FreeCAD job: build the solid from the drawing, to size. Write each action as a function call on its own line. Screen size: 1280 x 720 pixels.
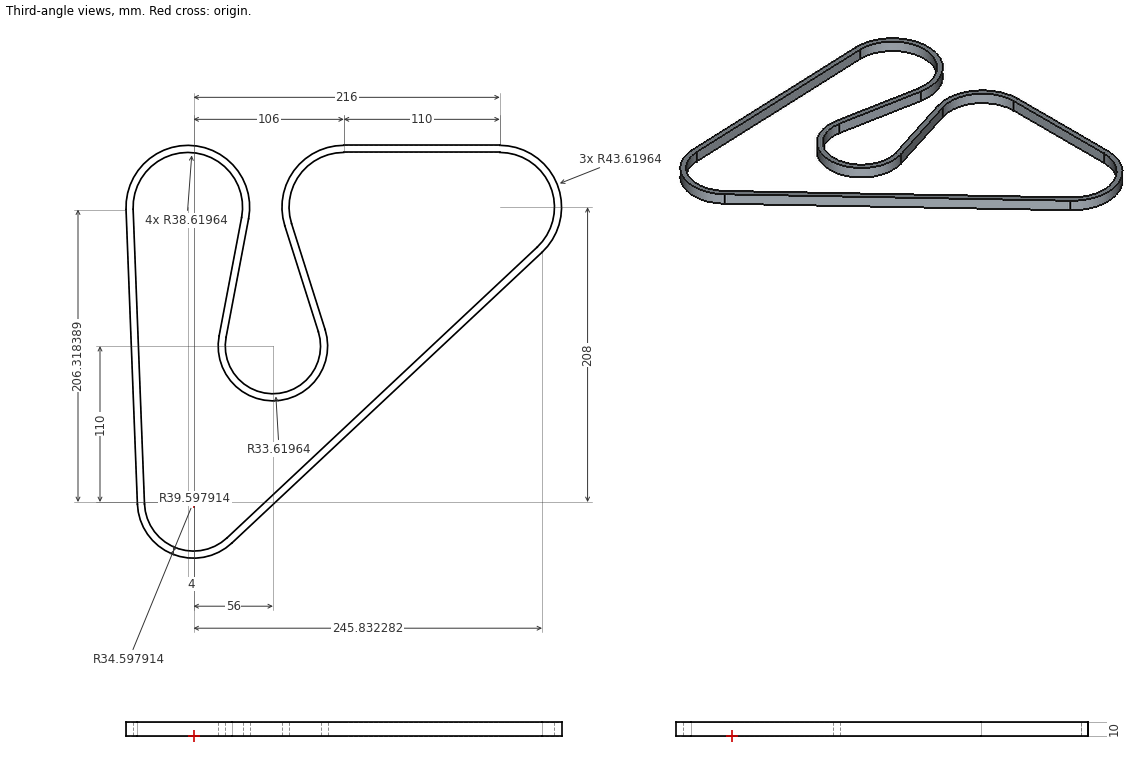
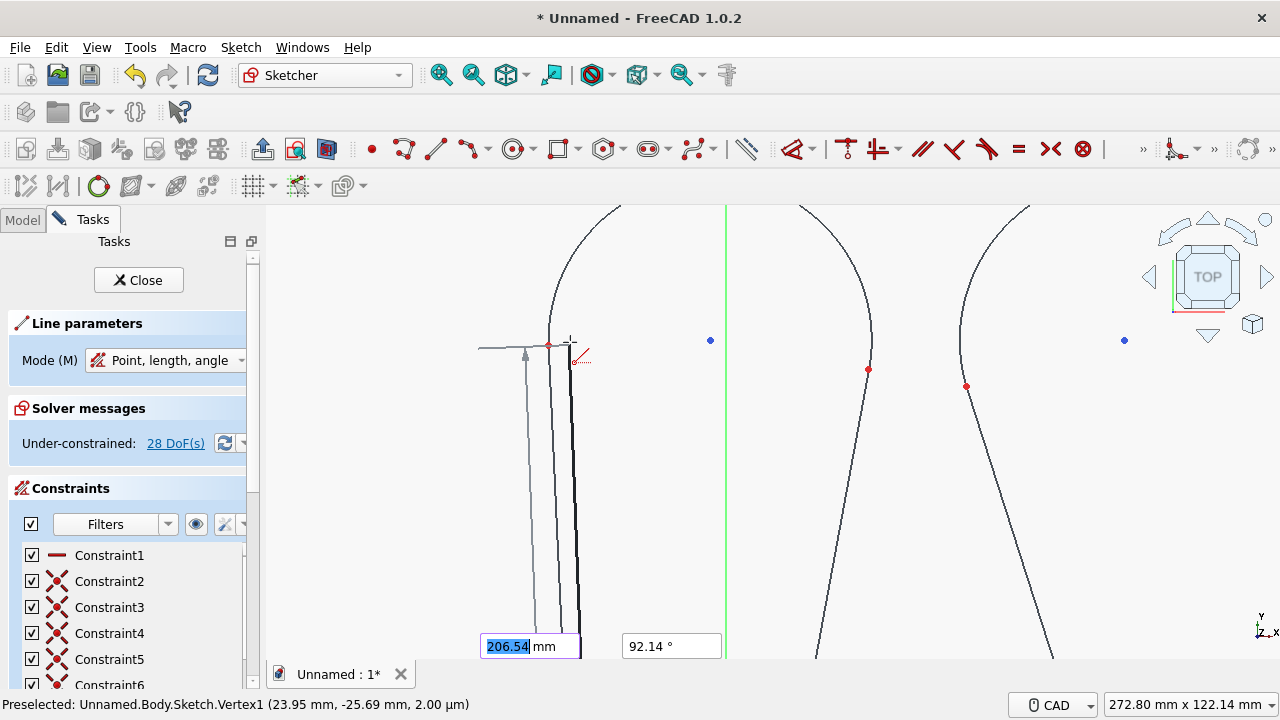
click(562, 339)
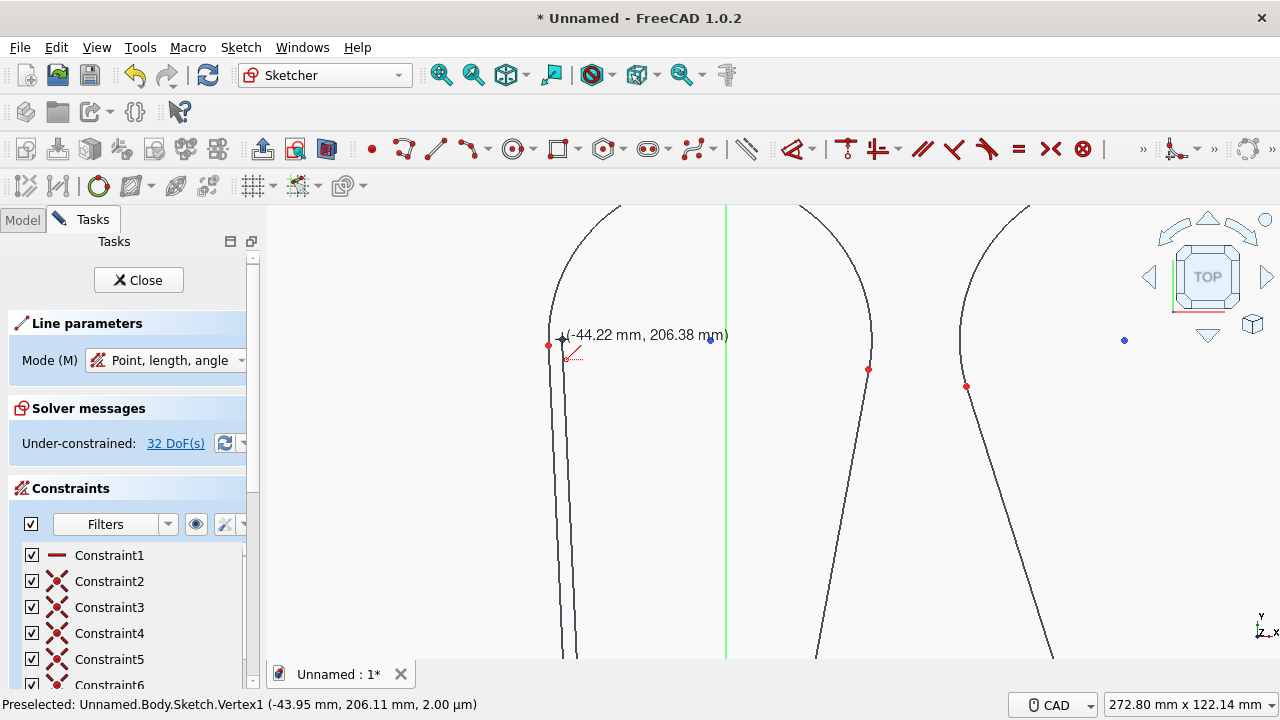
click(853, 361)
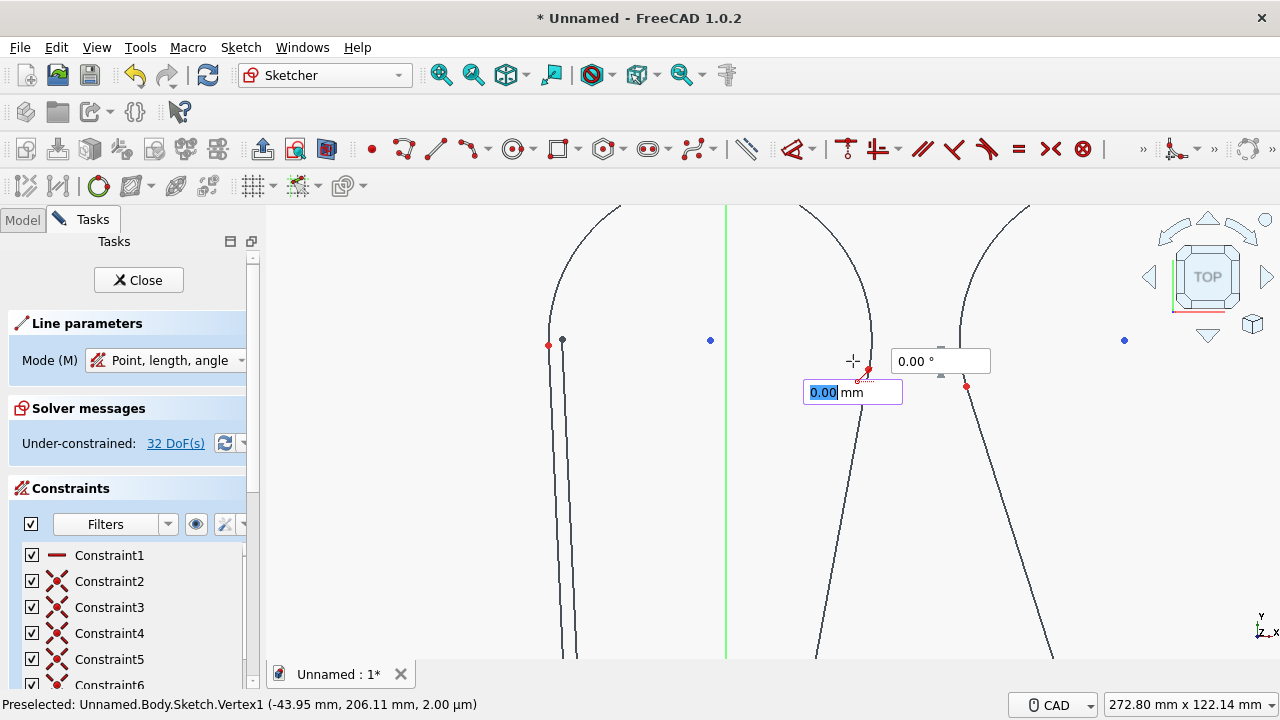
scroll(570, 342, down, 7)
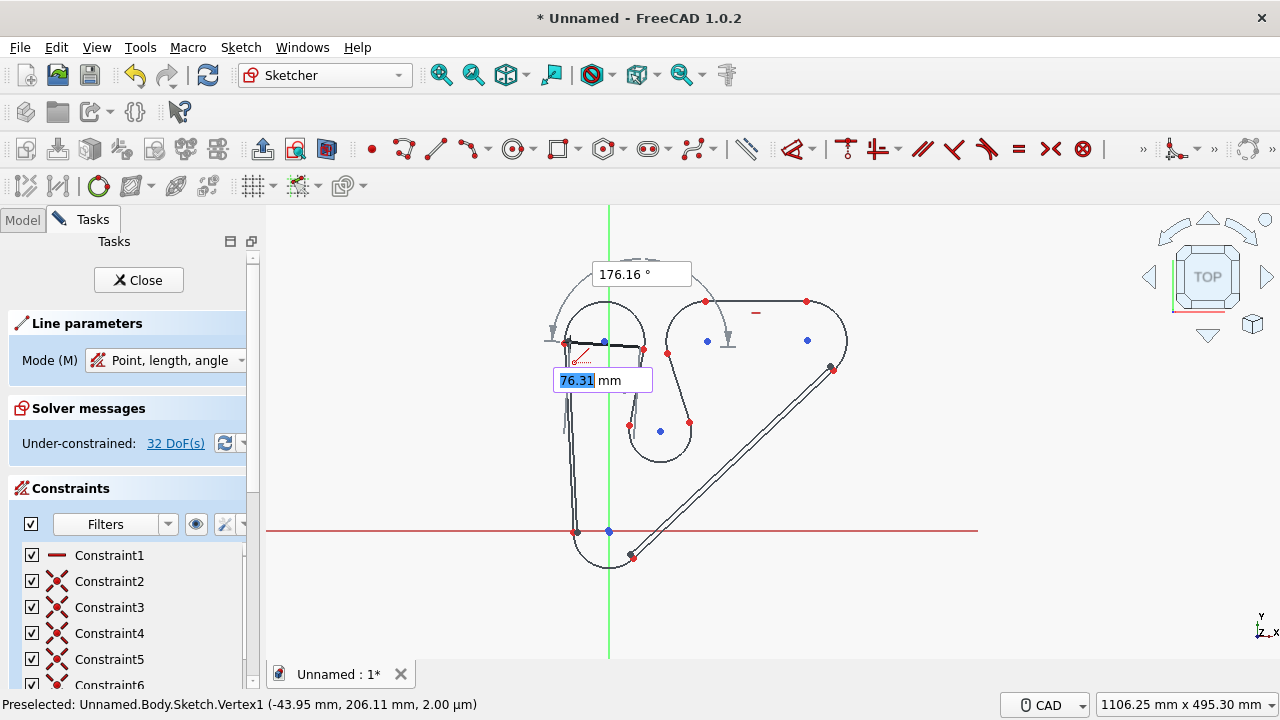
scroll(625, 423, up, 7)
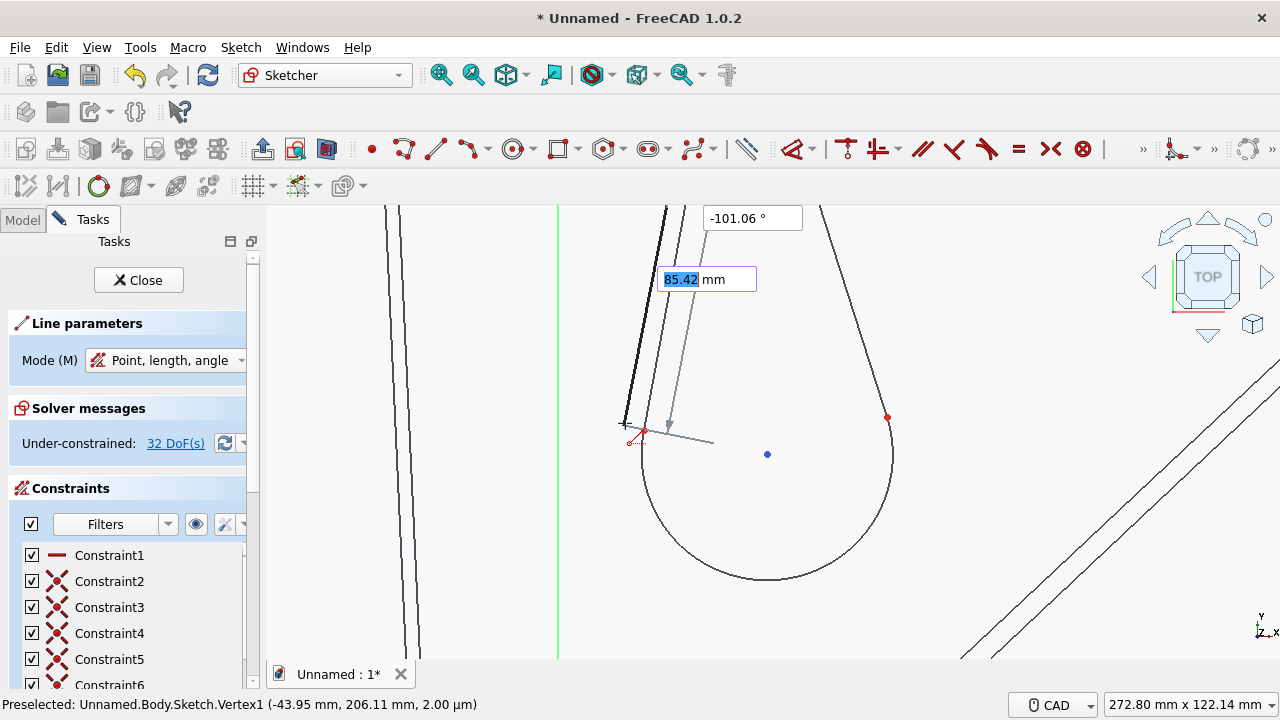
click(625, 423)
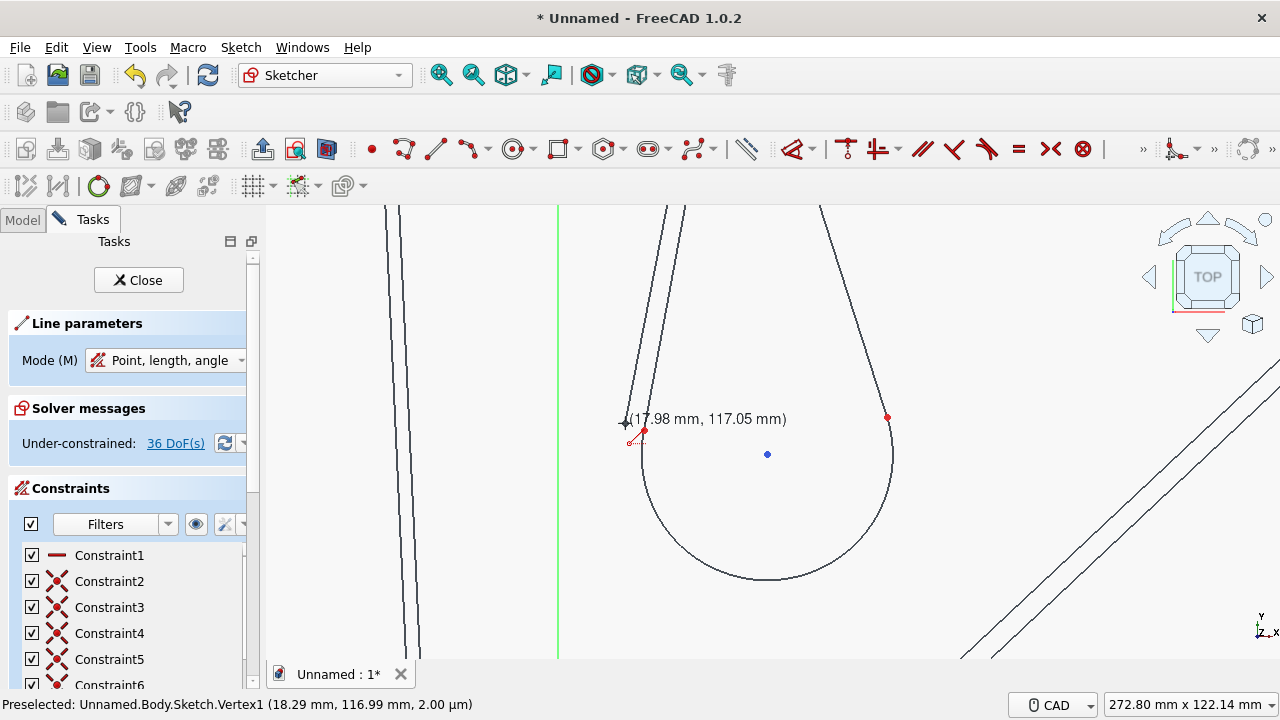
click(903, 407)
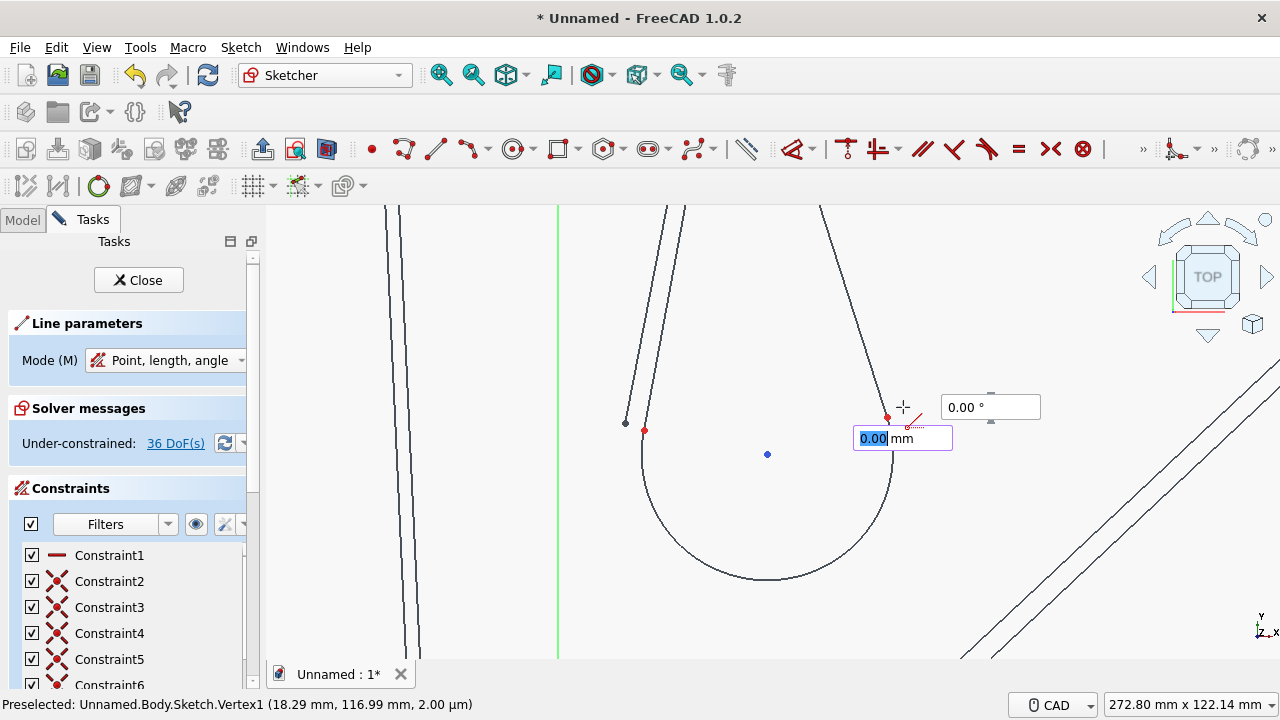
scroll(625, 423, down, 7)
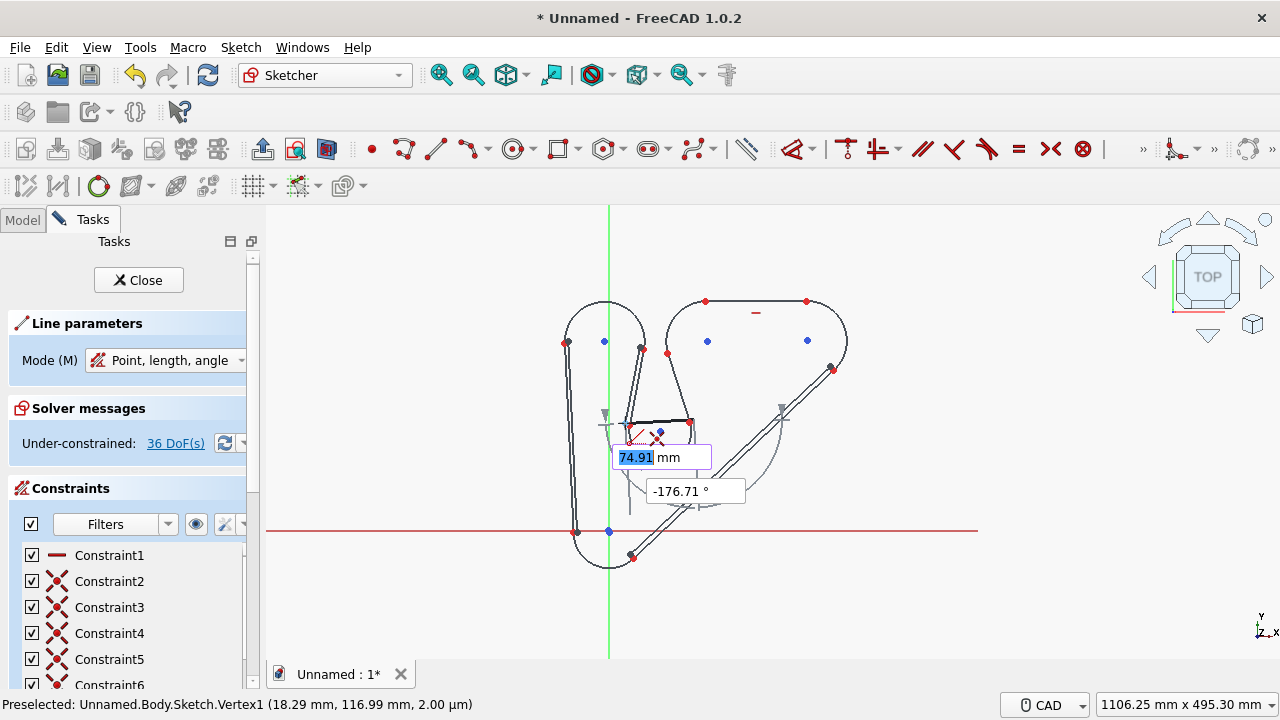
scroll(672, 351, up, 7)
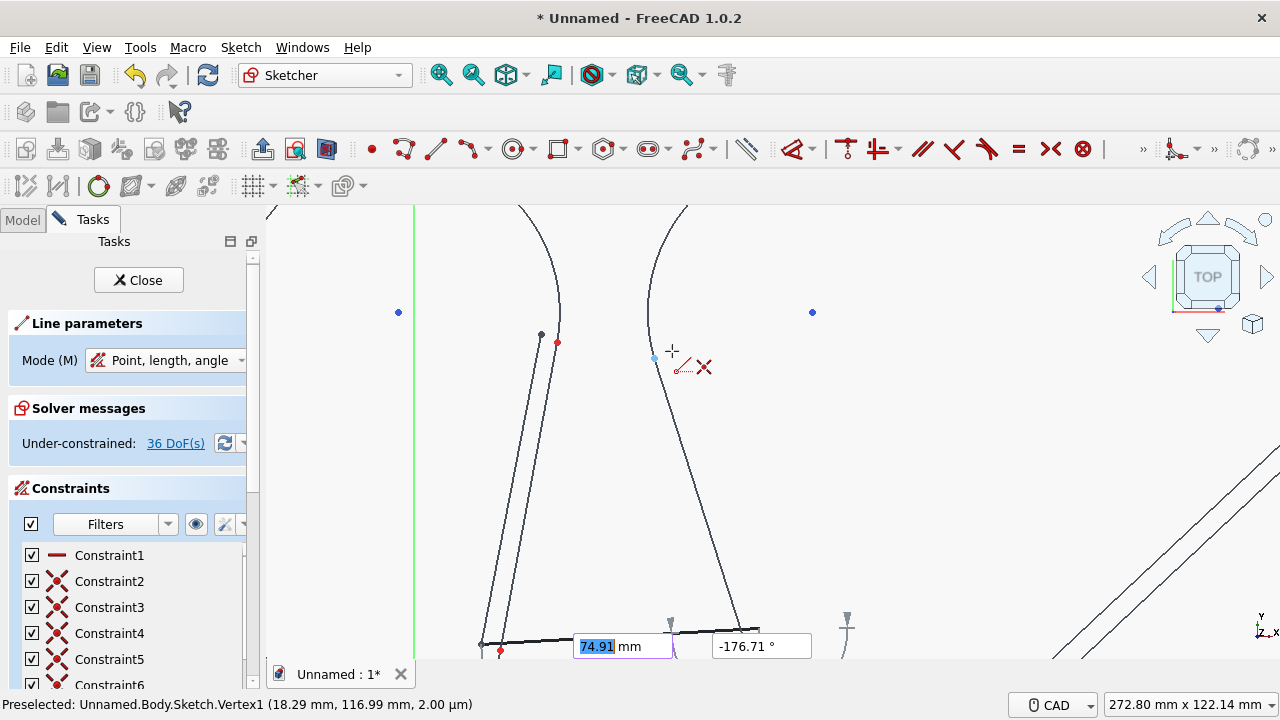
click(672, 350)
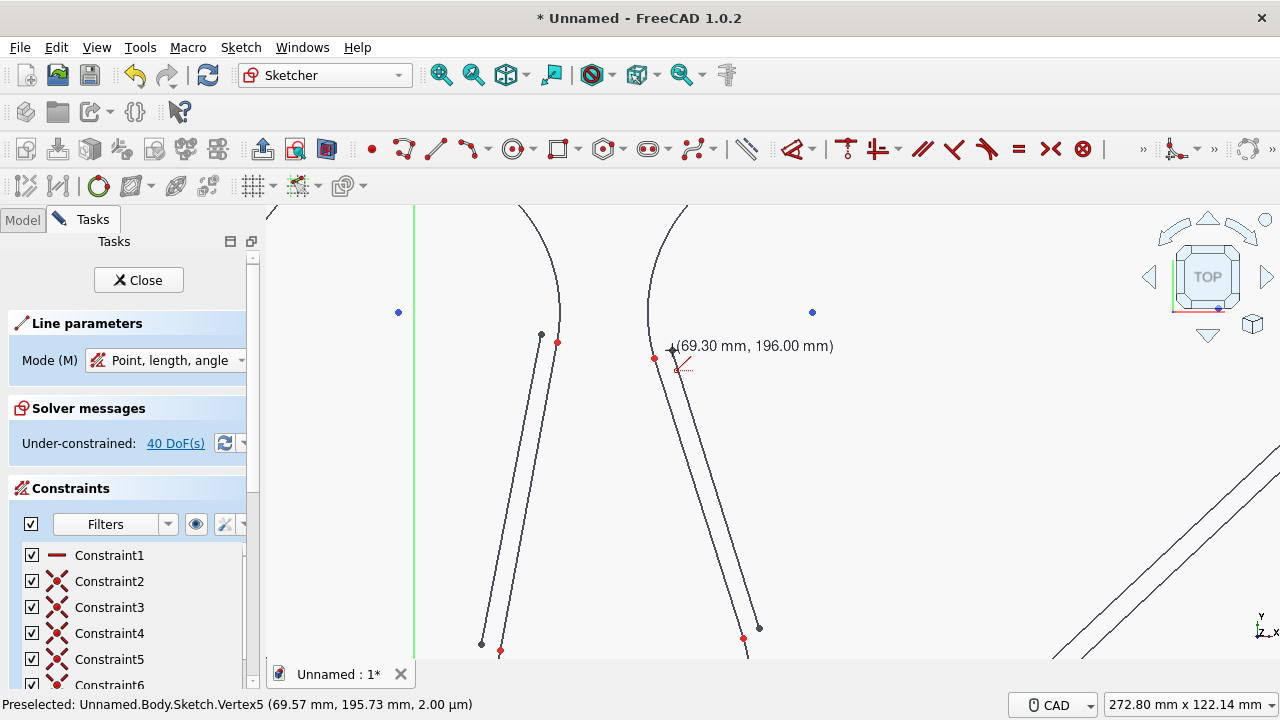
scroll(672, 351, down, 7)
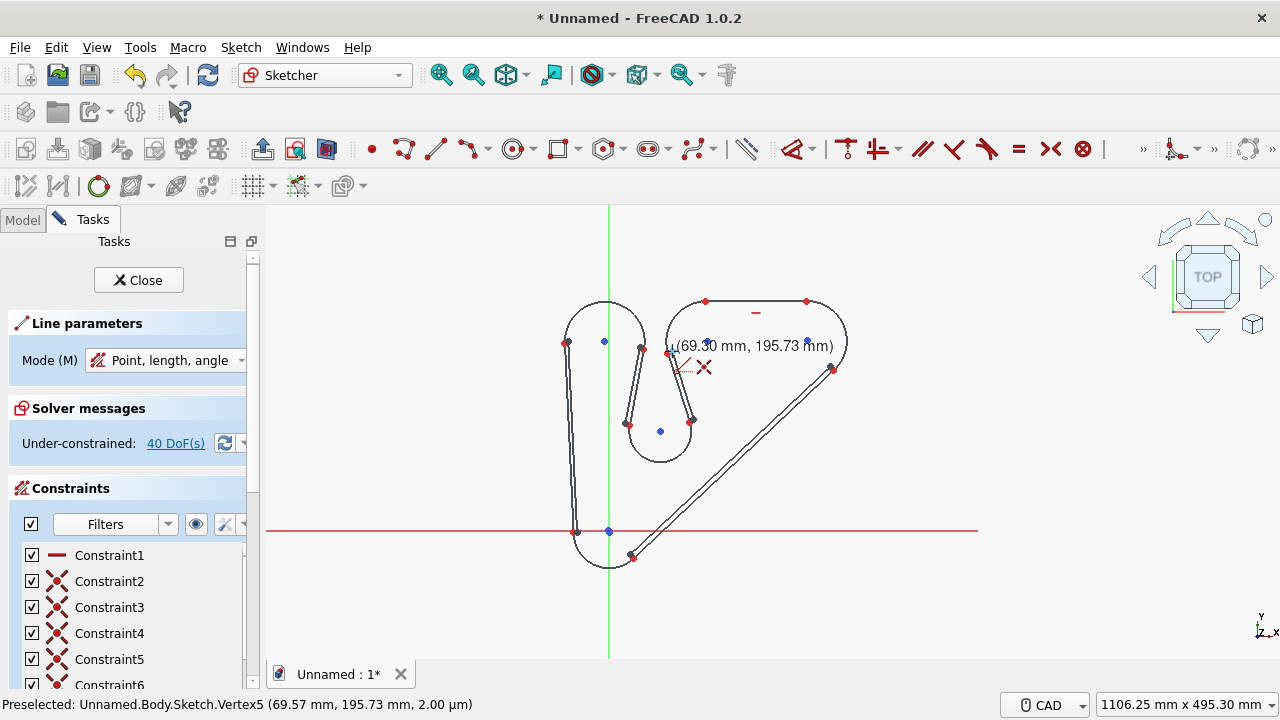
scroll(706, 305, up, 7)